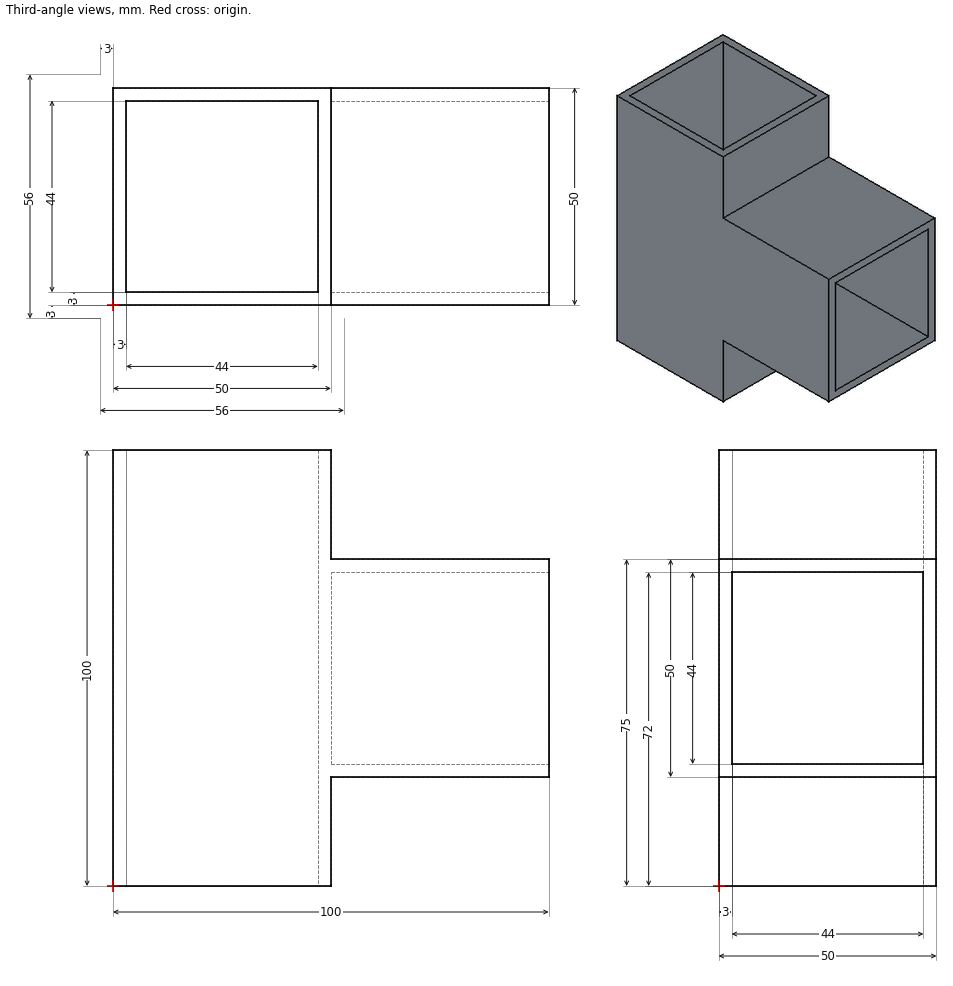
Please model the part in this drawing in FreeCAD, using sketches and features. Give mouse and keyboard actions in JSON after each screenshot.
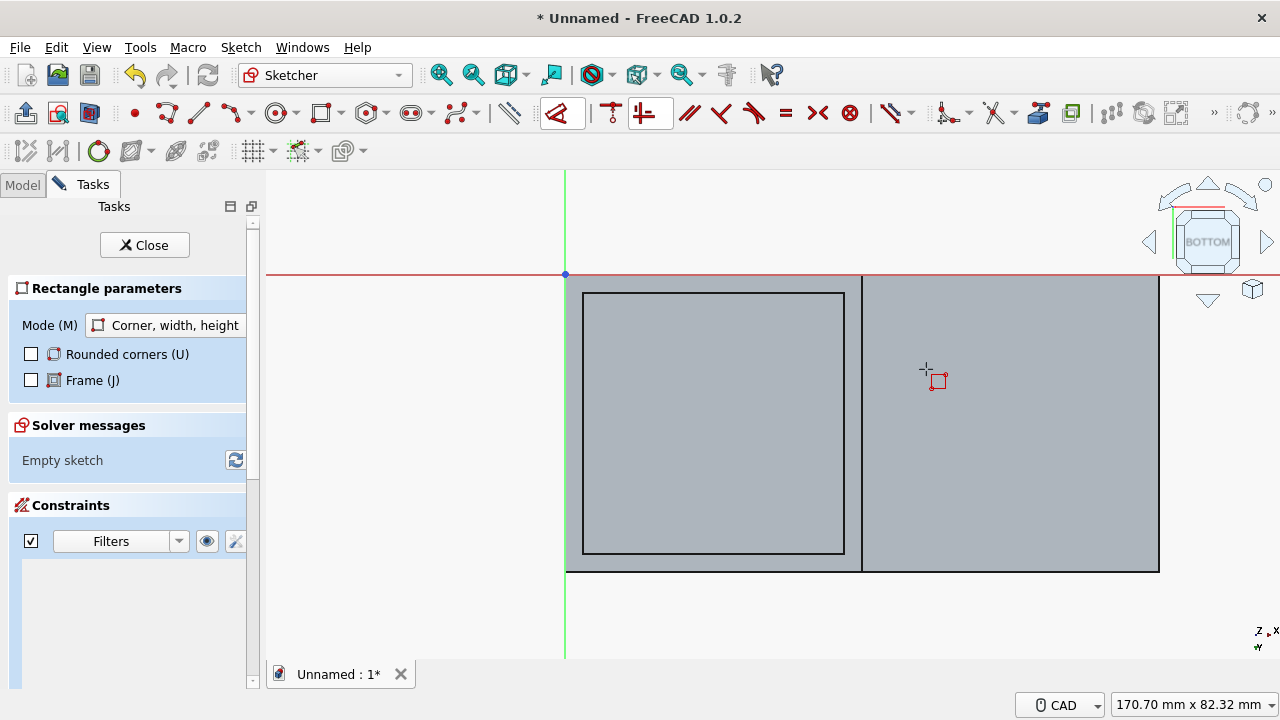
{"action": "left_click", "coordinate": [583, 293]}
{"action": "left_click", "coordinate": [844, 554]}
{"action": "key", "text": "Escape"}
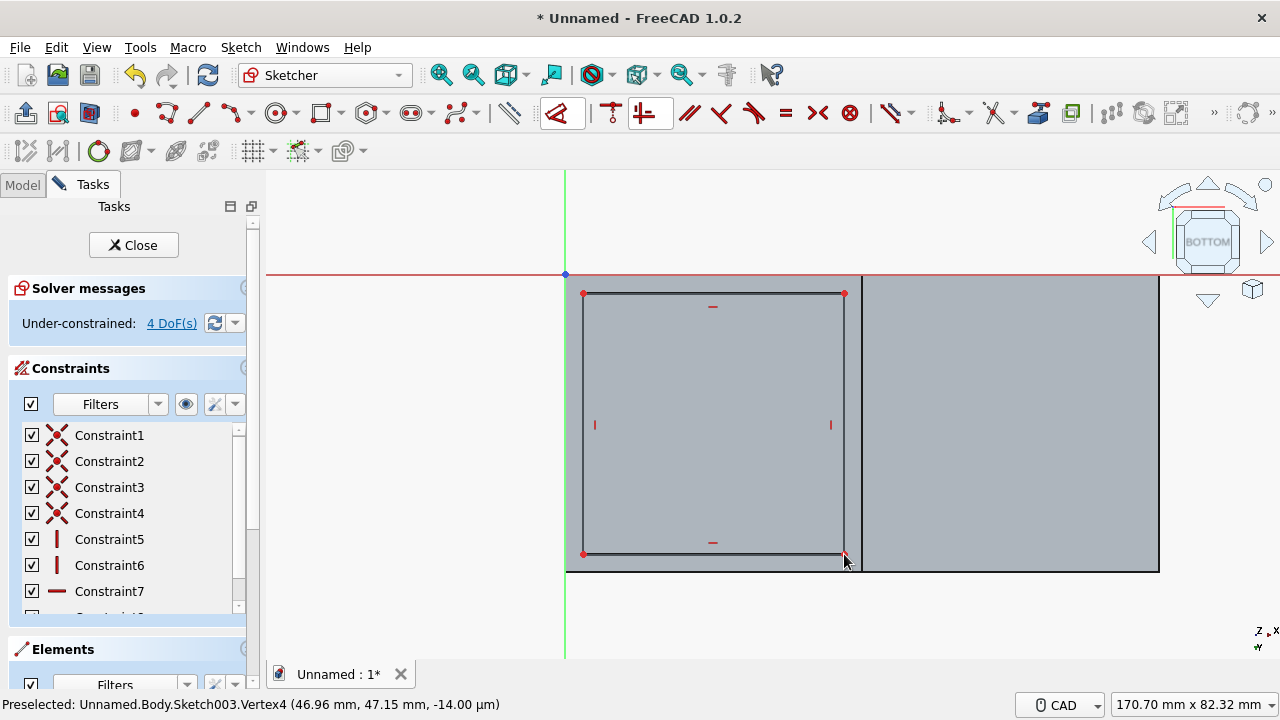
{"action": "left_click", "coordinate": [583, 372]}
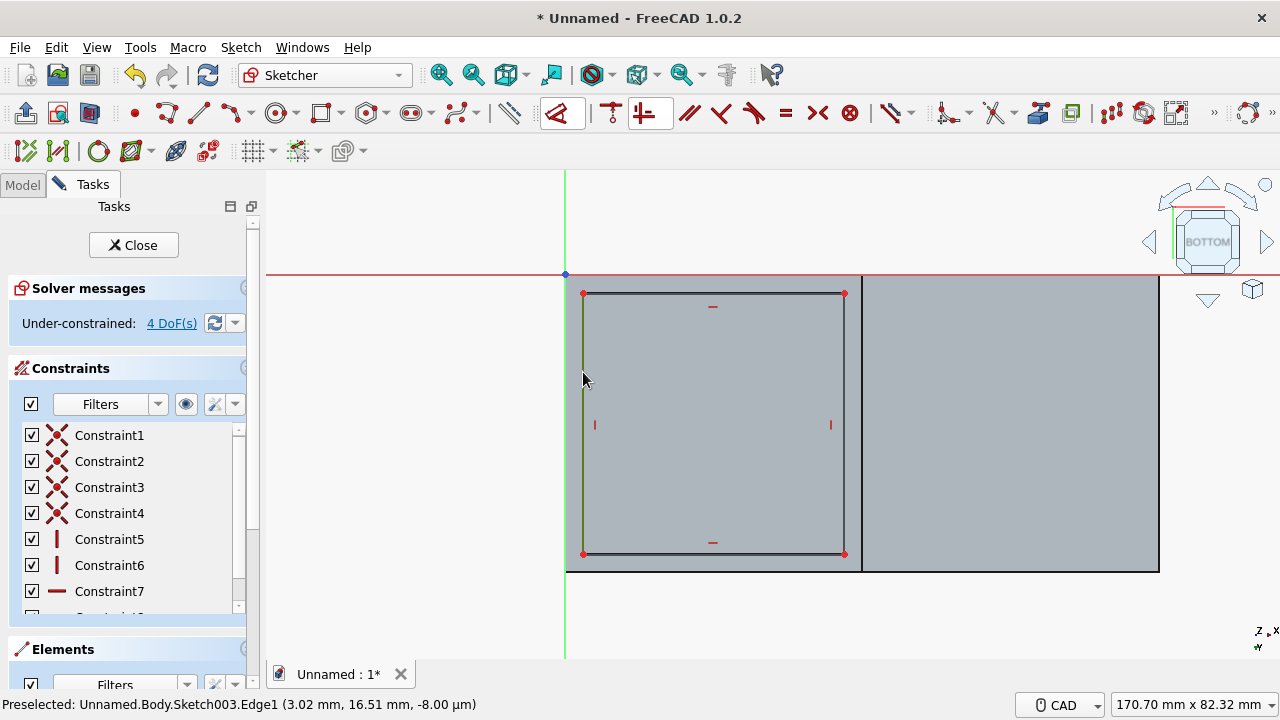
{"action": "left_click", "coordinate": [580, 114]}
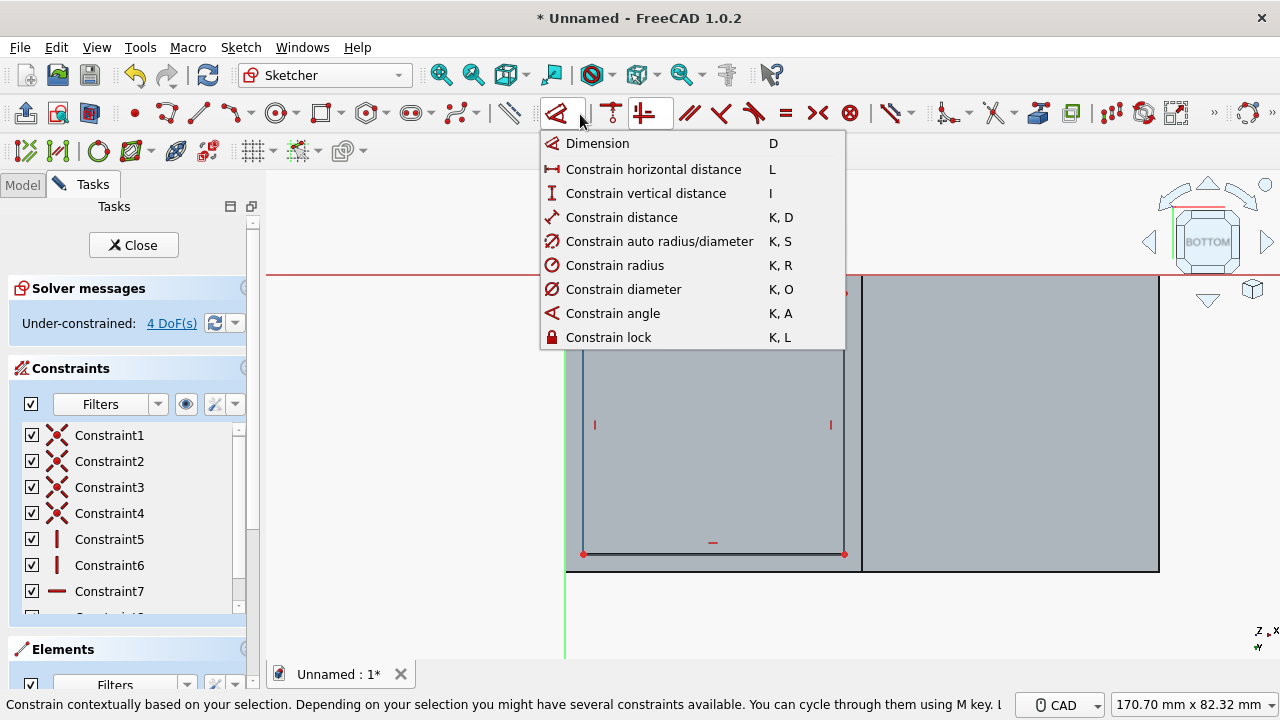
{"action": "left_click", "coordinate": [693, 193]}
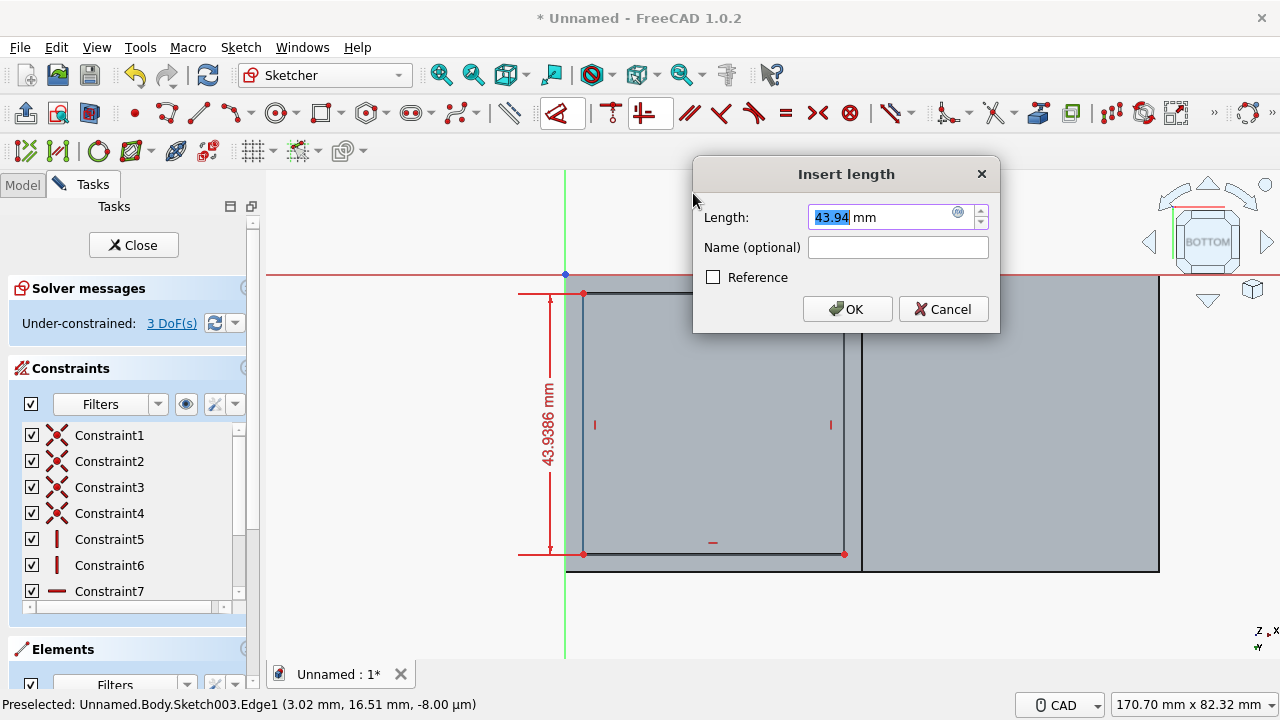
{"action": "type", "text": "44"}
{"action": "key", "text": "Return"}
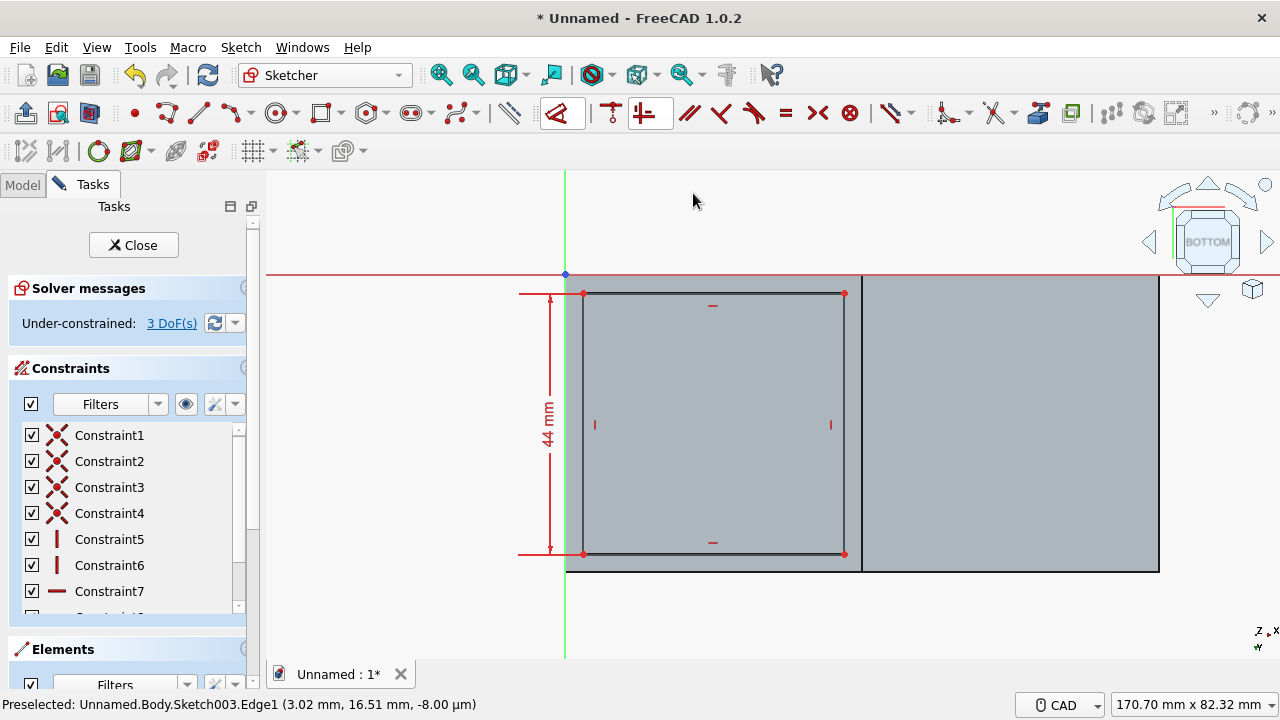
{"action": "left_click", "coordinate": [661, 555]}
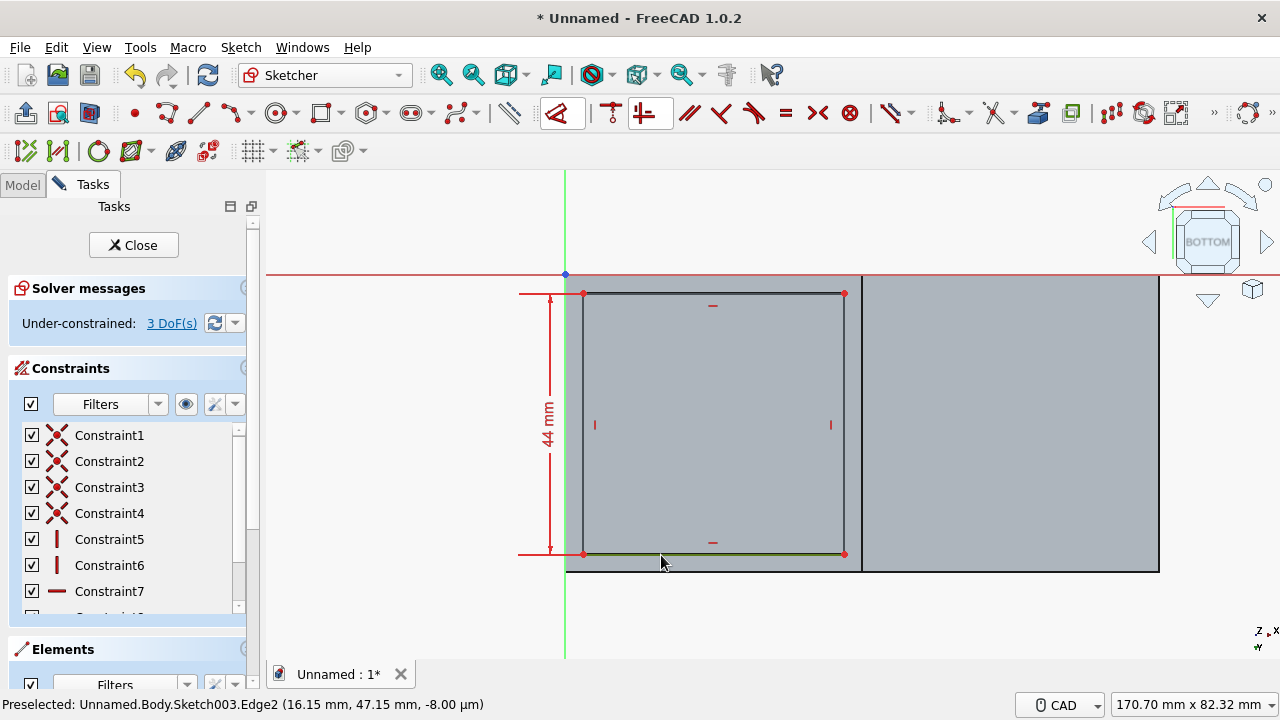
{"action": "key", "text": "l"}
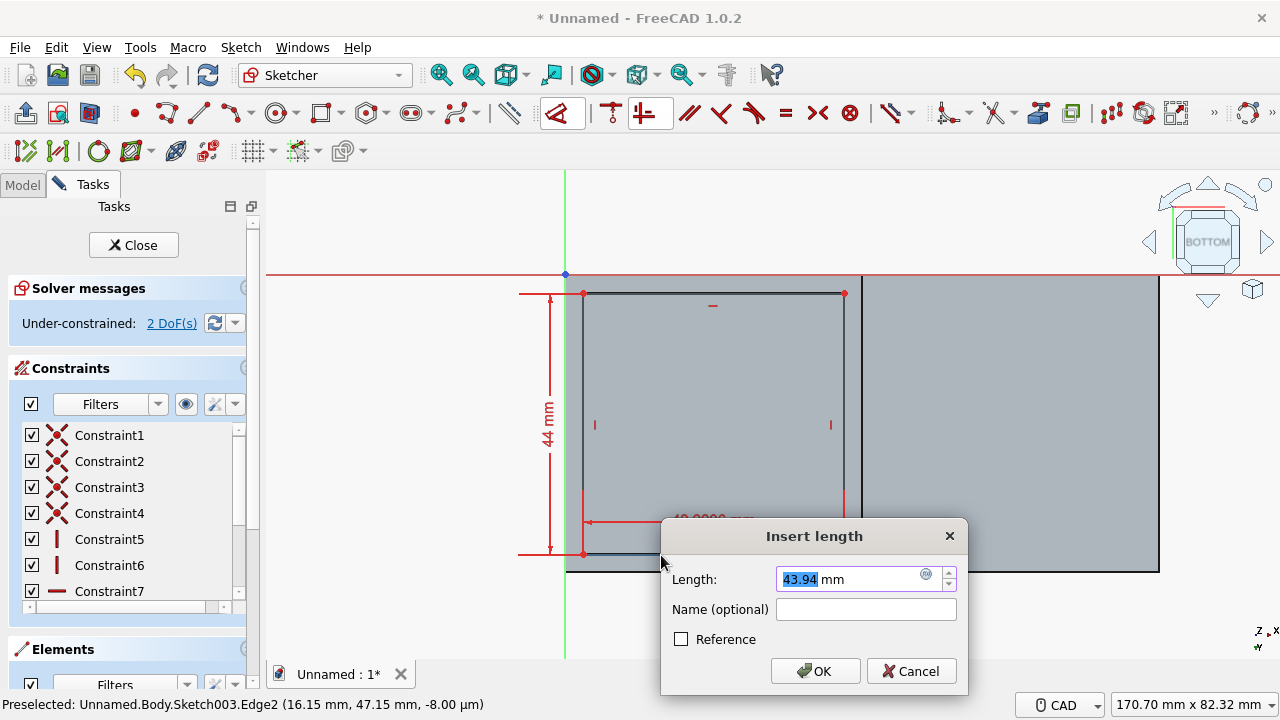
{"action": "type", "text": "44"}
{"action": "key", "text": "Return"}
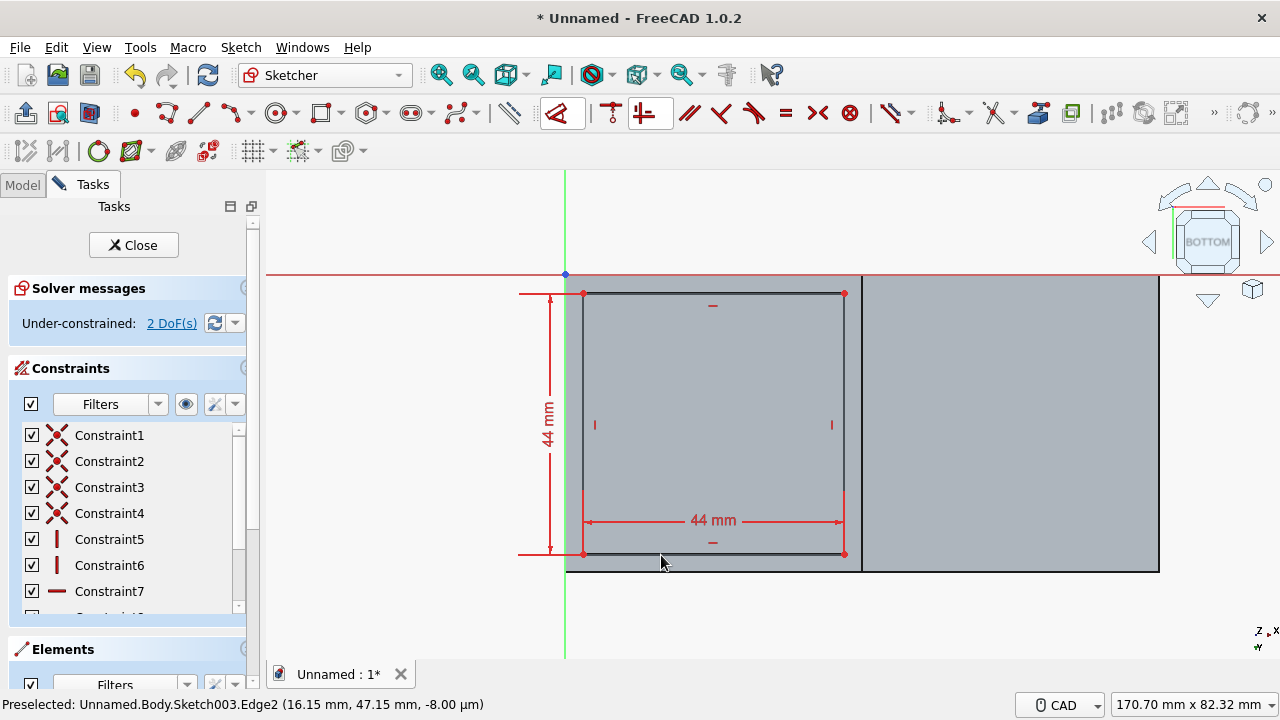
{"action": "scroll", "coordinate": [583, 294], "scroll_direction": "up", "scroll_amount": 5}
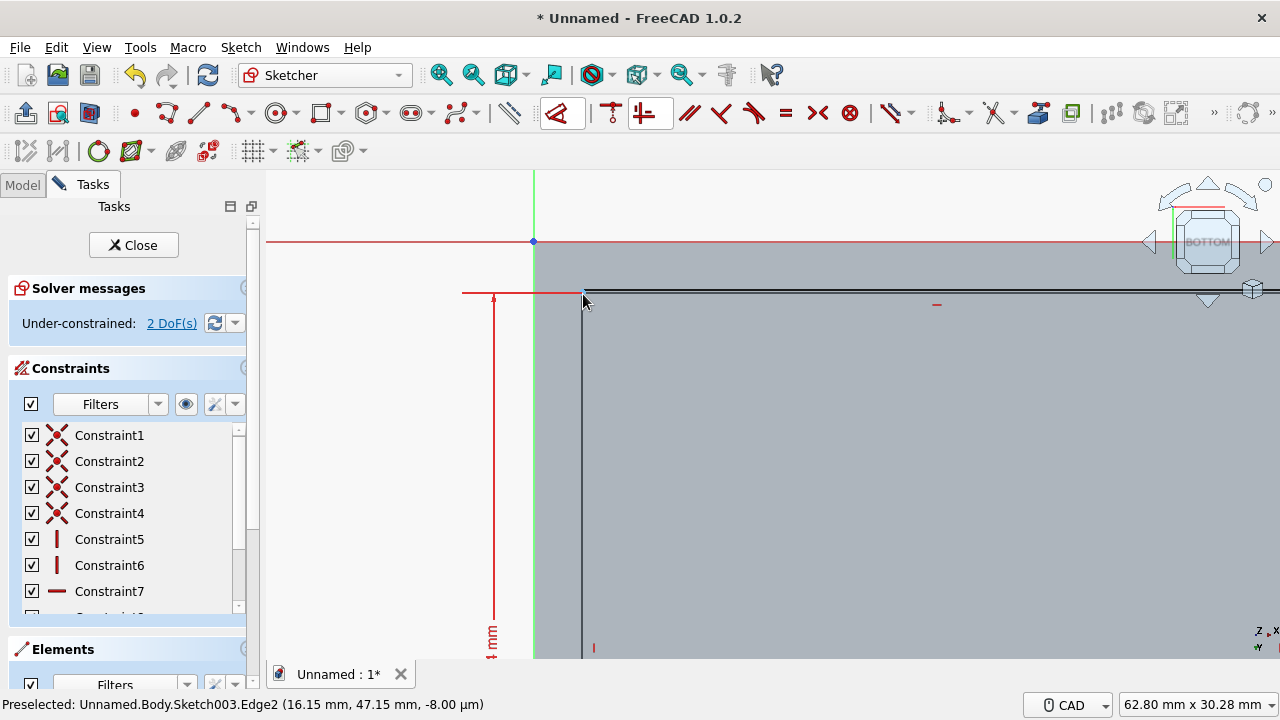
{"action": "left_click", "coordinate": [582, 293]}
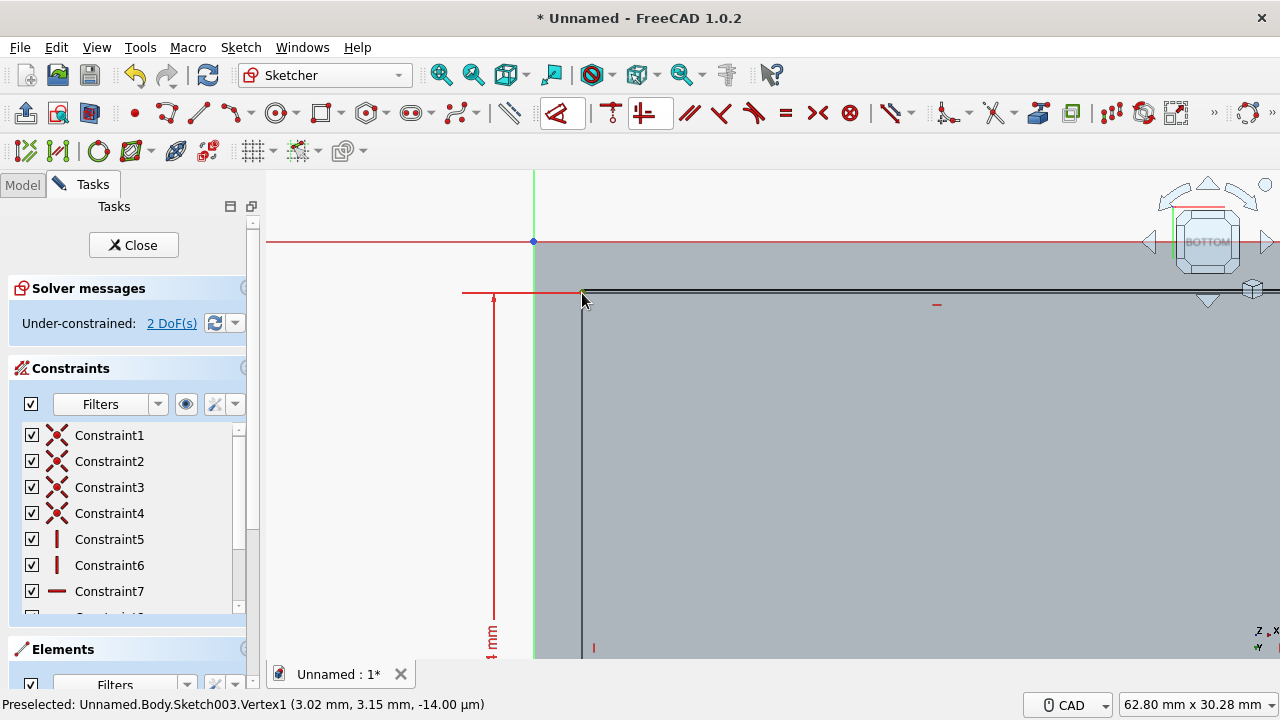
{"action": "key", "text": "l"}